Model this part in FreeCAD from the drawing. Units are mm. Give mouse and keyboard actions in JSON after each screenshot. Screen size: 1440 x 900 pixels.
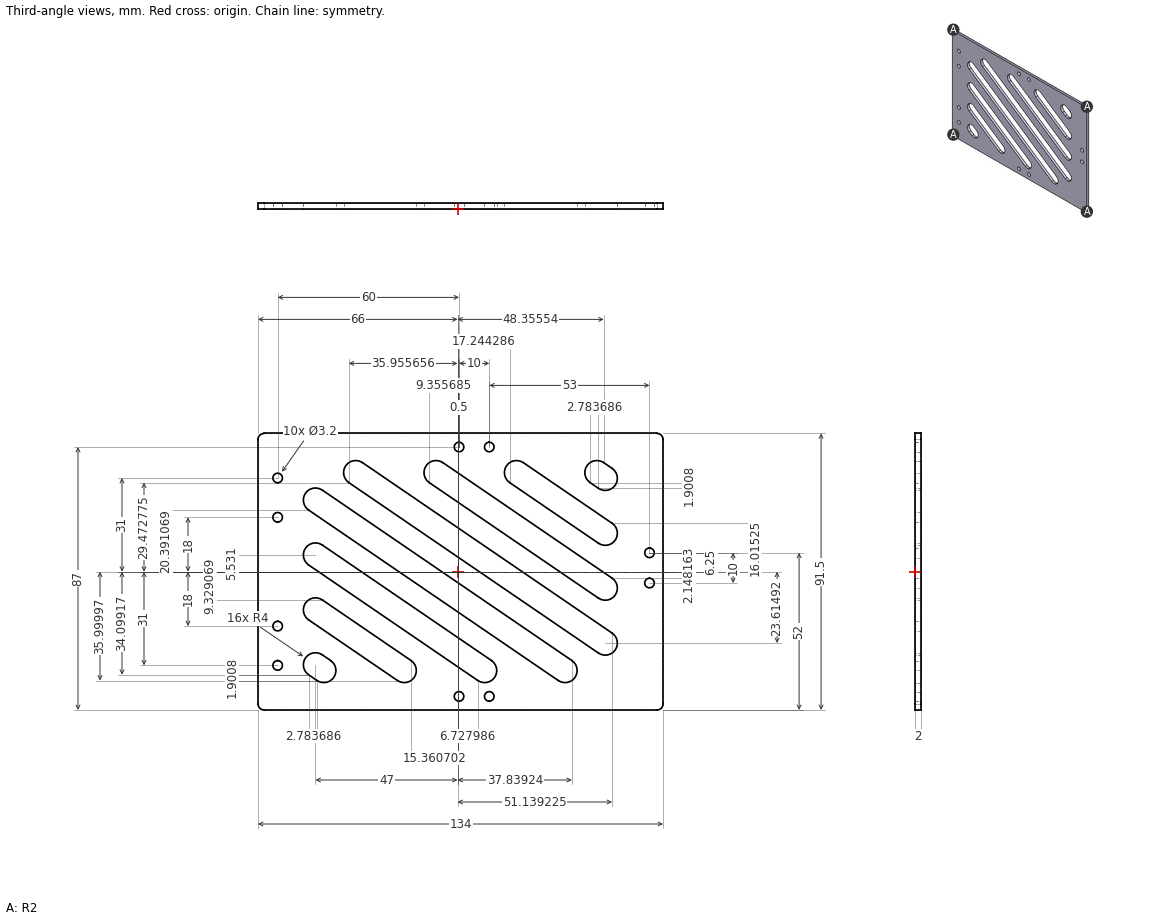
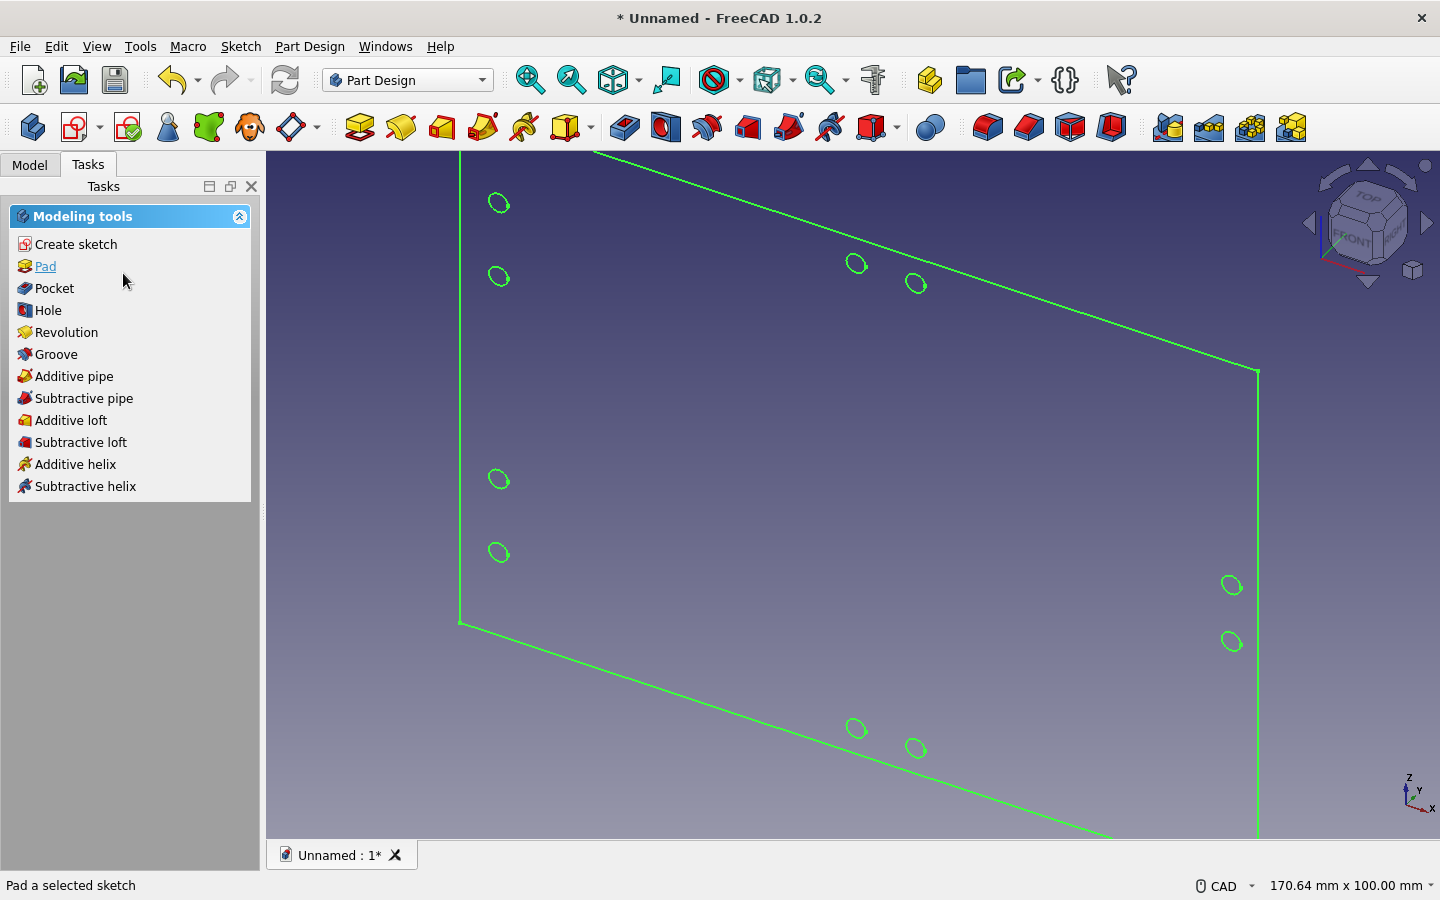
{"action": "left_click", "coordinate": [360, 128]}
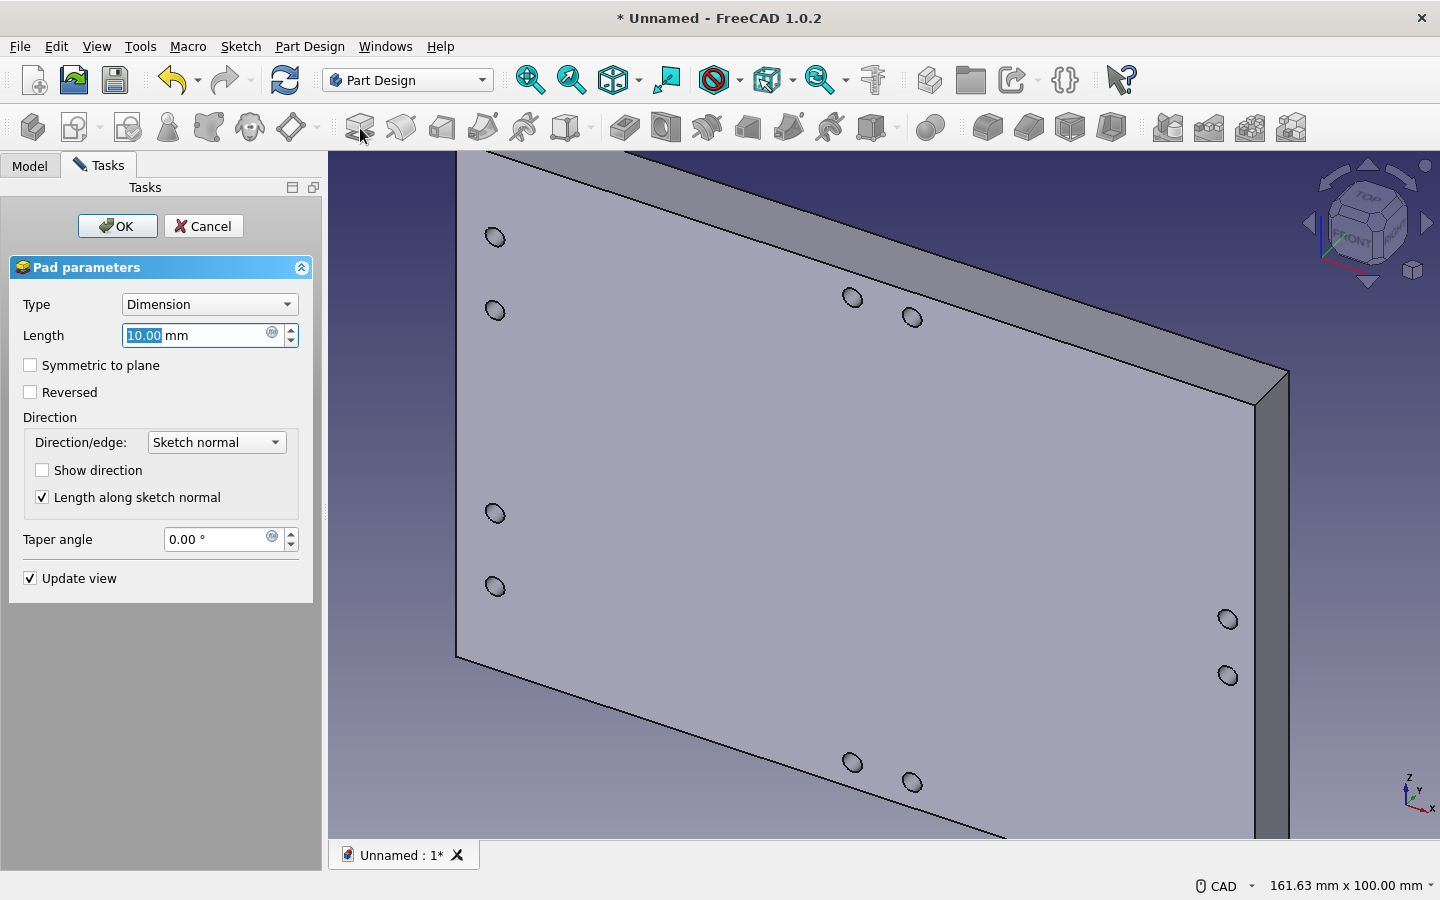
{"action": "type", "text": "2"}
{"action": "key", "text": "Tab"}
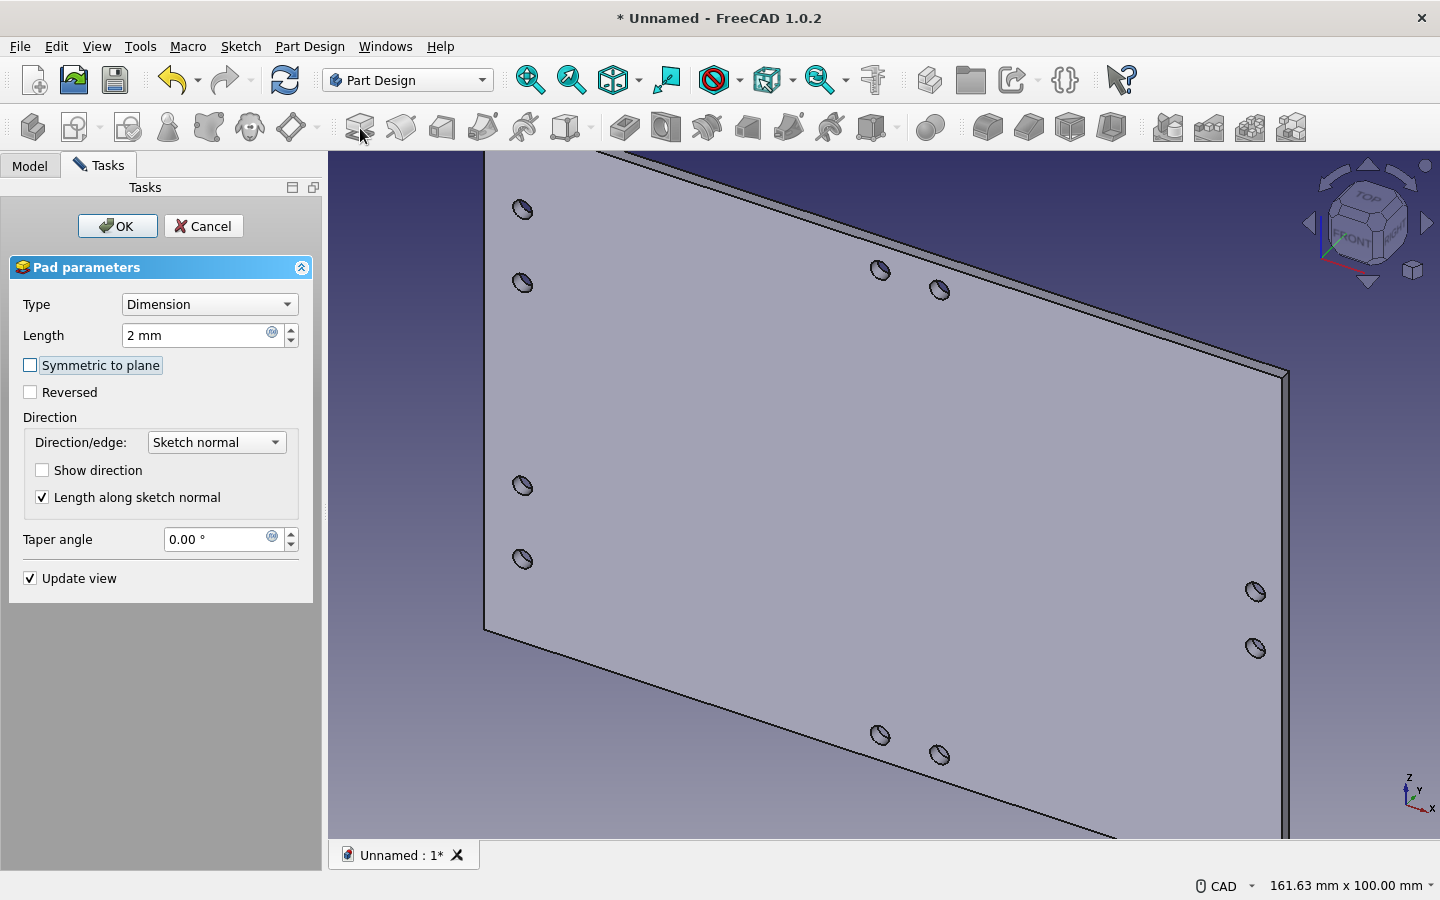
{"action": "left_click", "coordinate": [31, 392]}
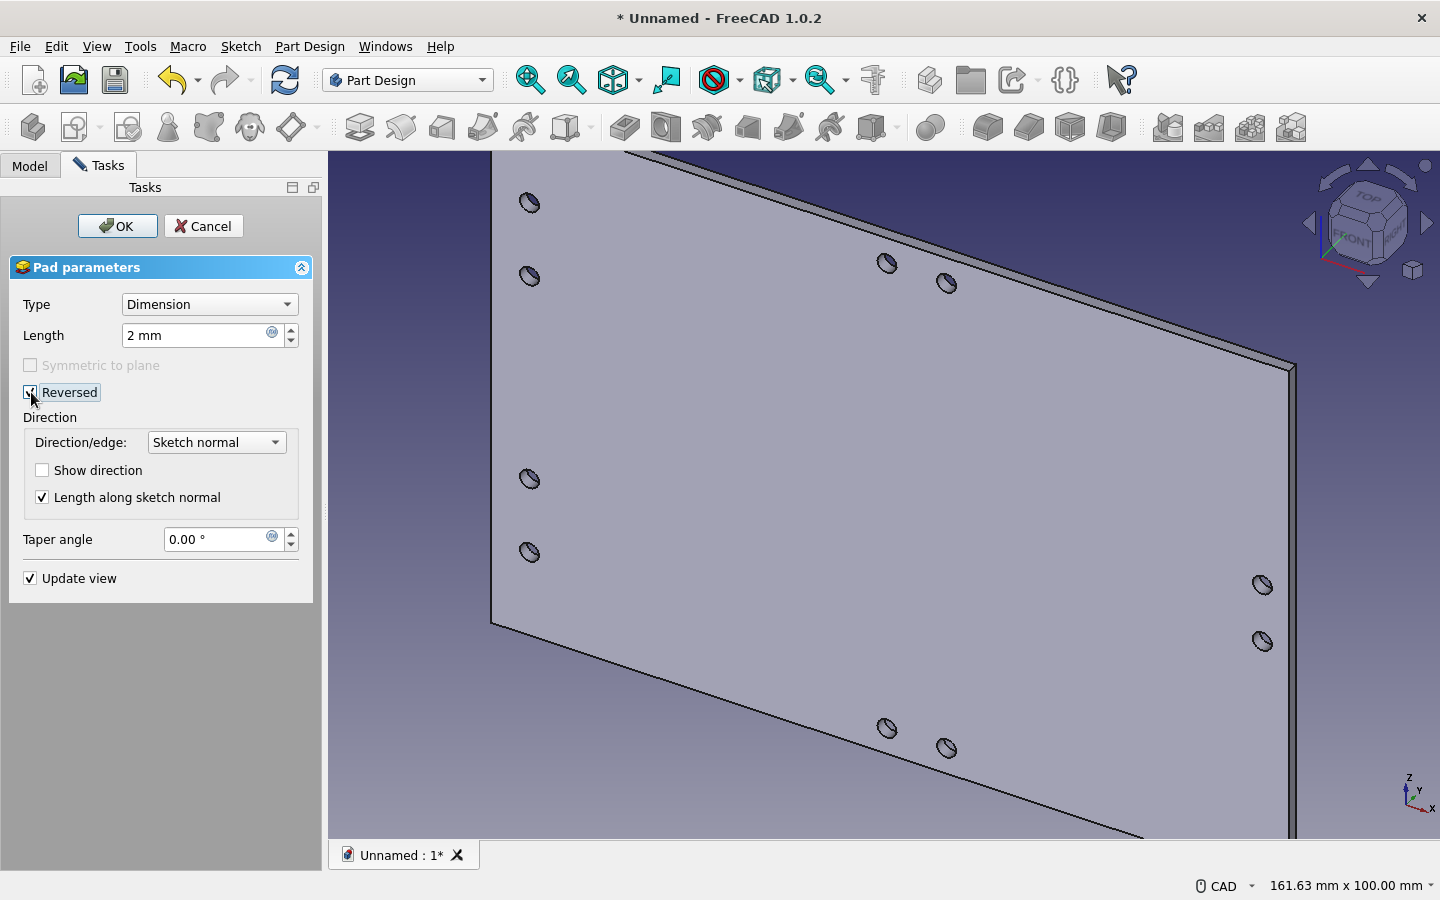
{"action": "left_click", "coordinate": [118, 226]}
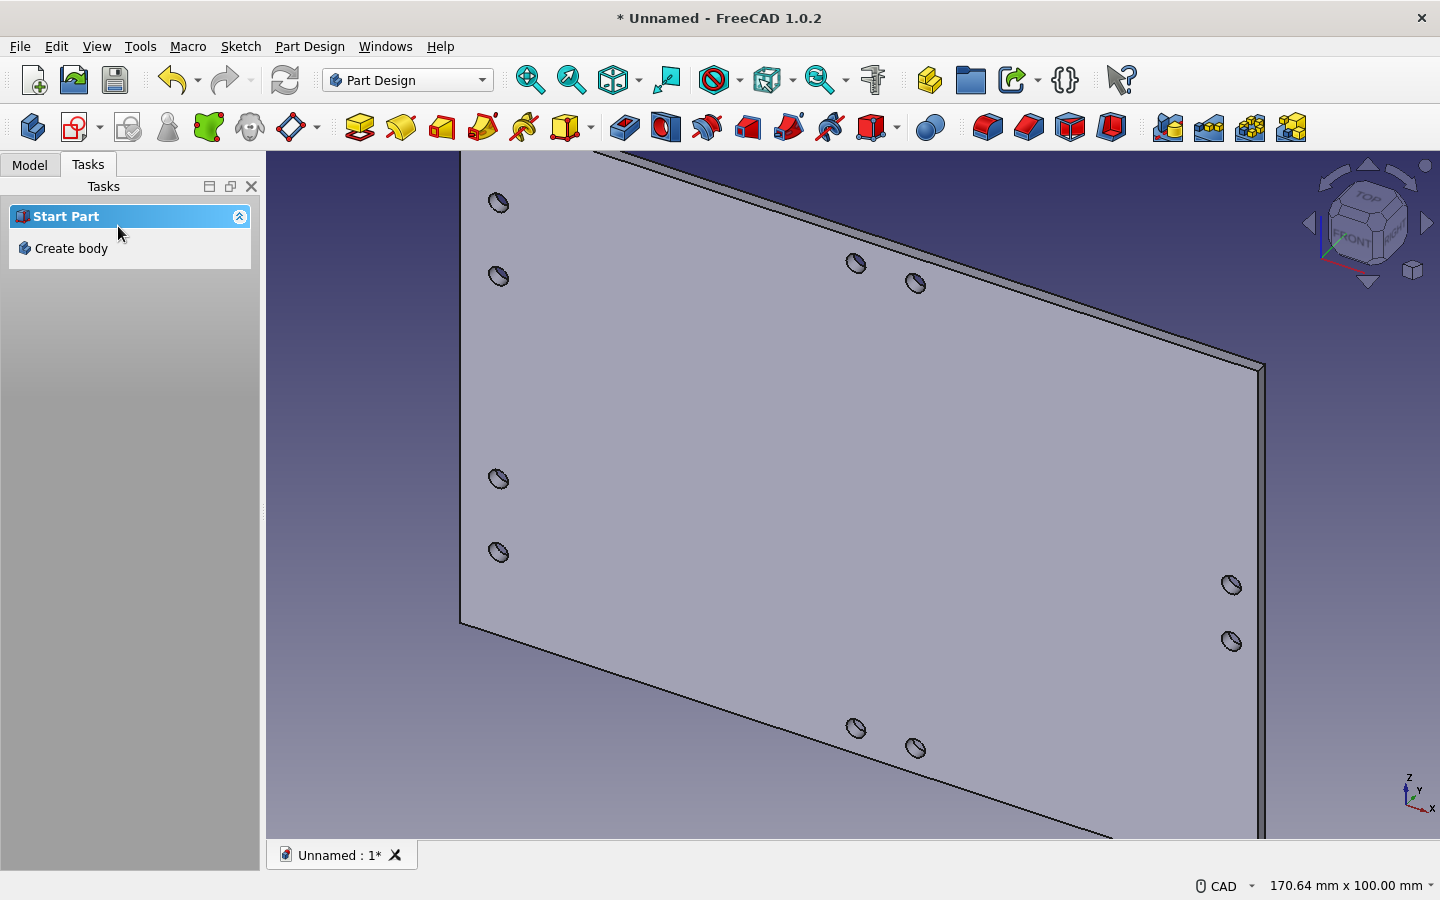
{"action": "left_click", "coordinate": [531, 80]}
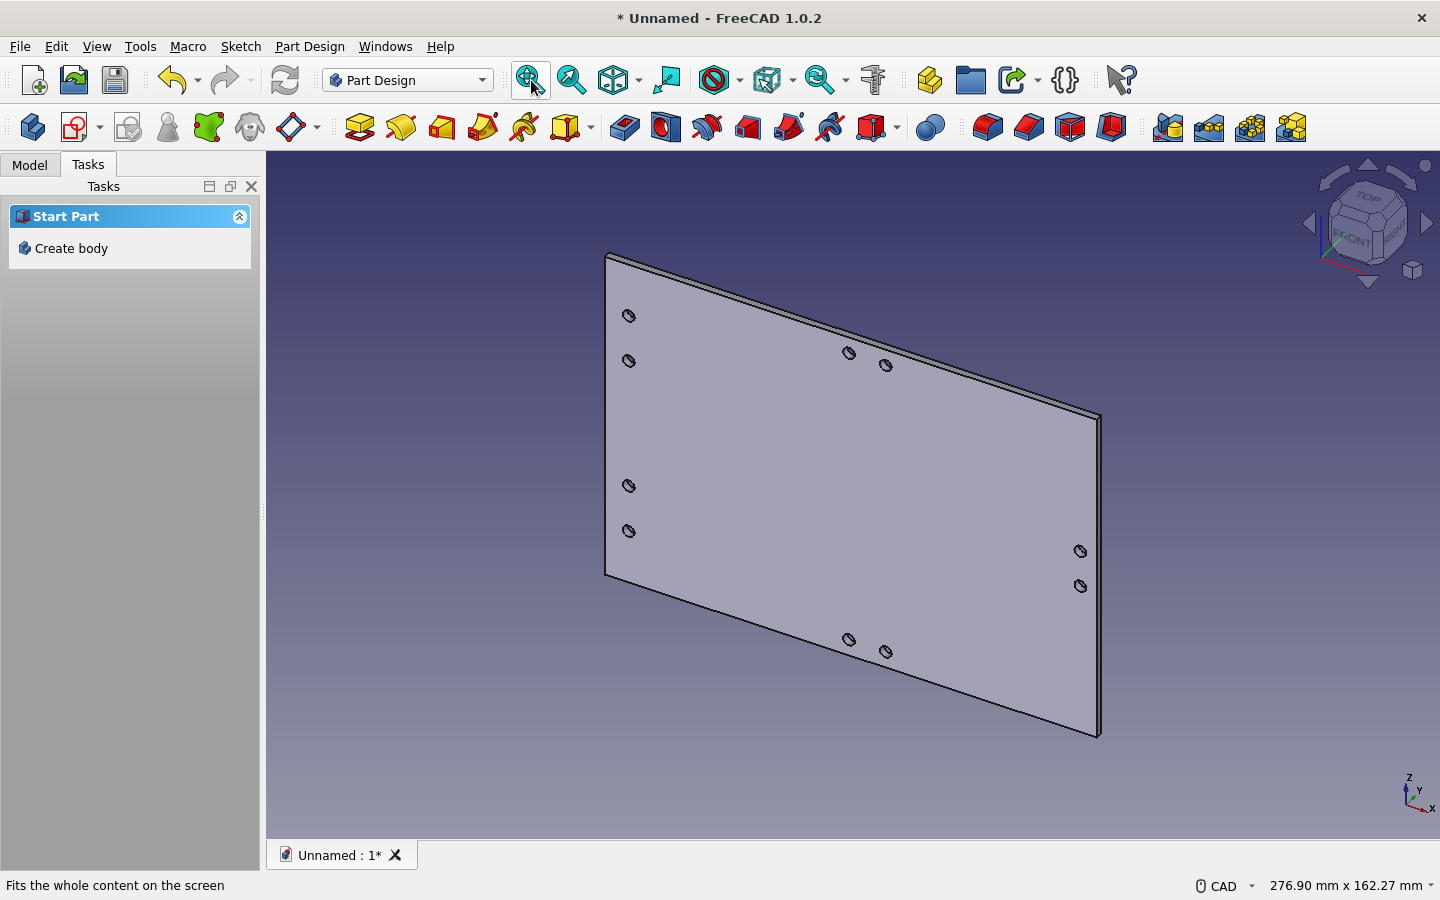
{"action": "key", "text": "4"}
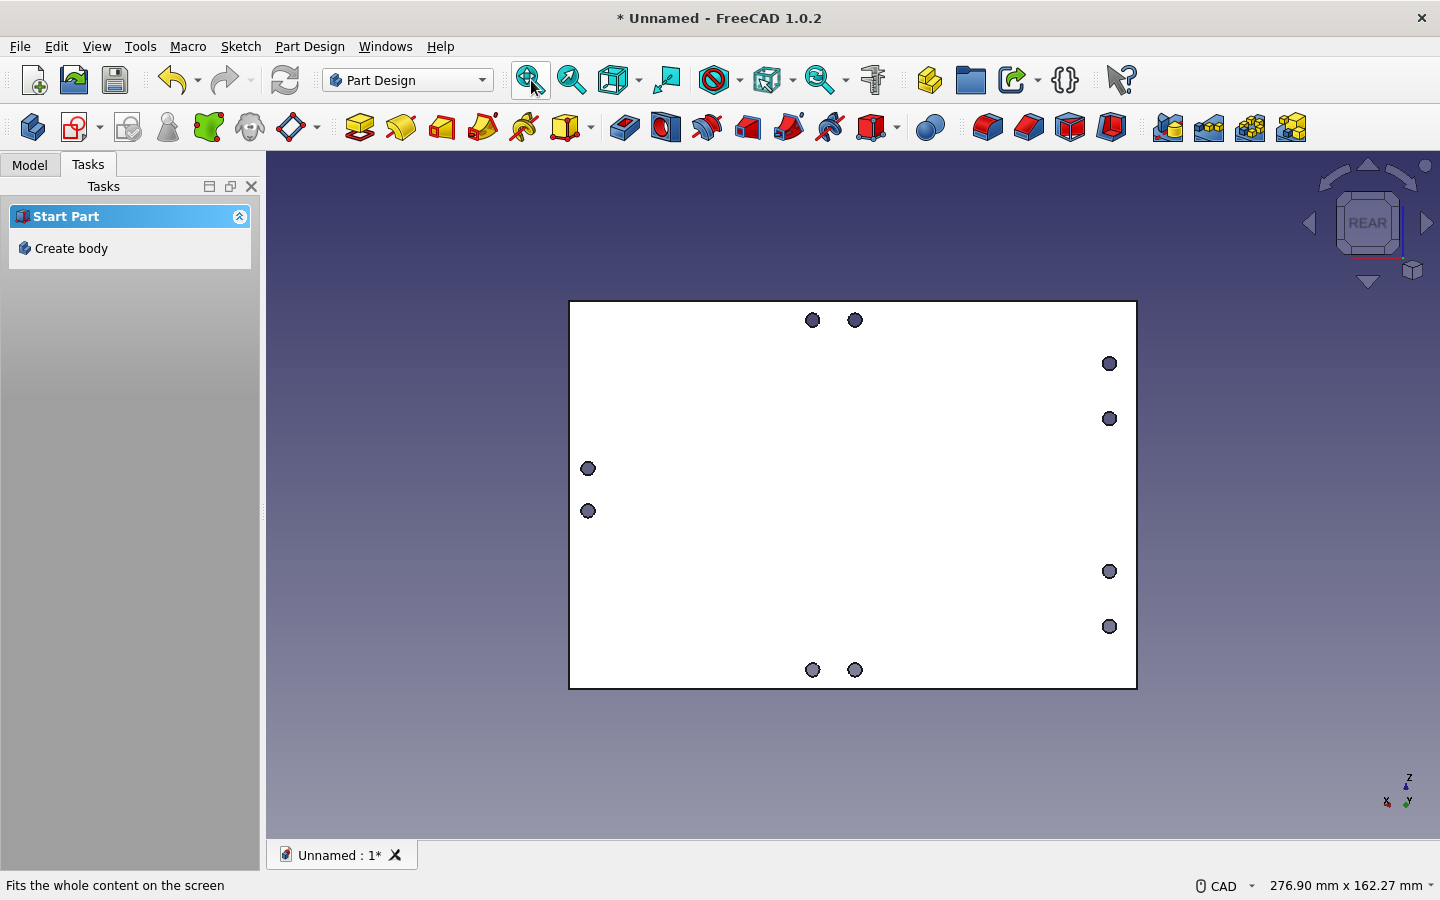
{"action": "left_click", "coordinate": [934, 494]}